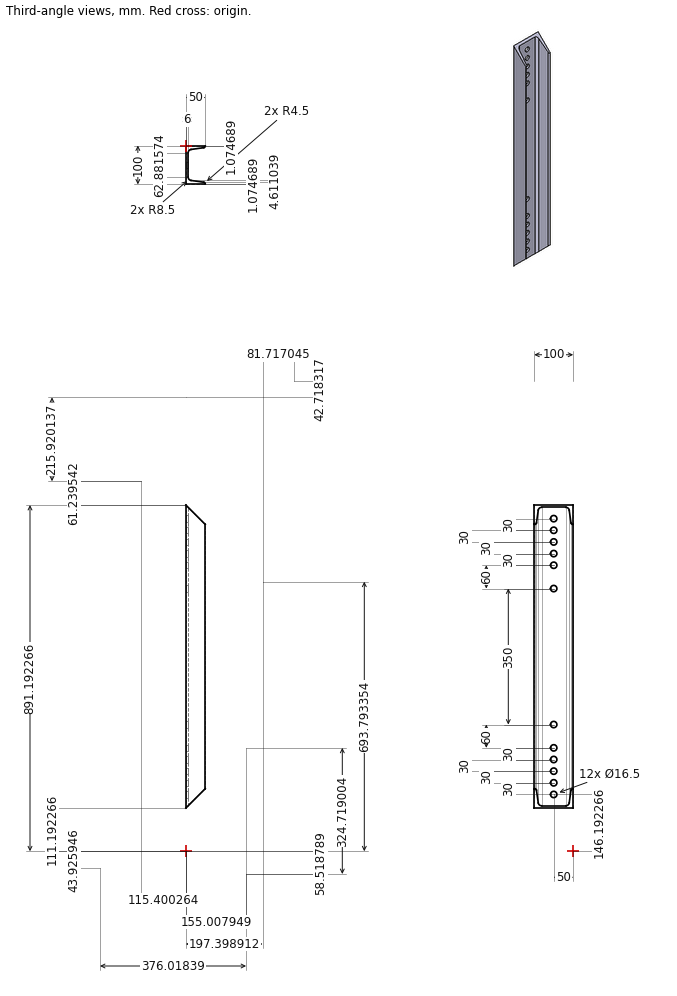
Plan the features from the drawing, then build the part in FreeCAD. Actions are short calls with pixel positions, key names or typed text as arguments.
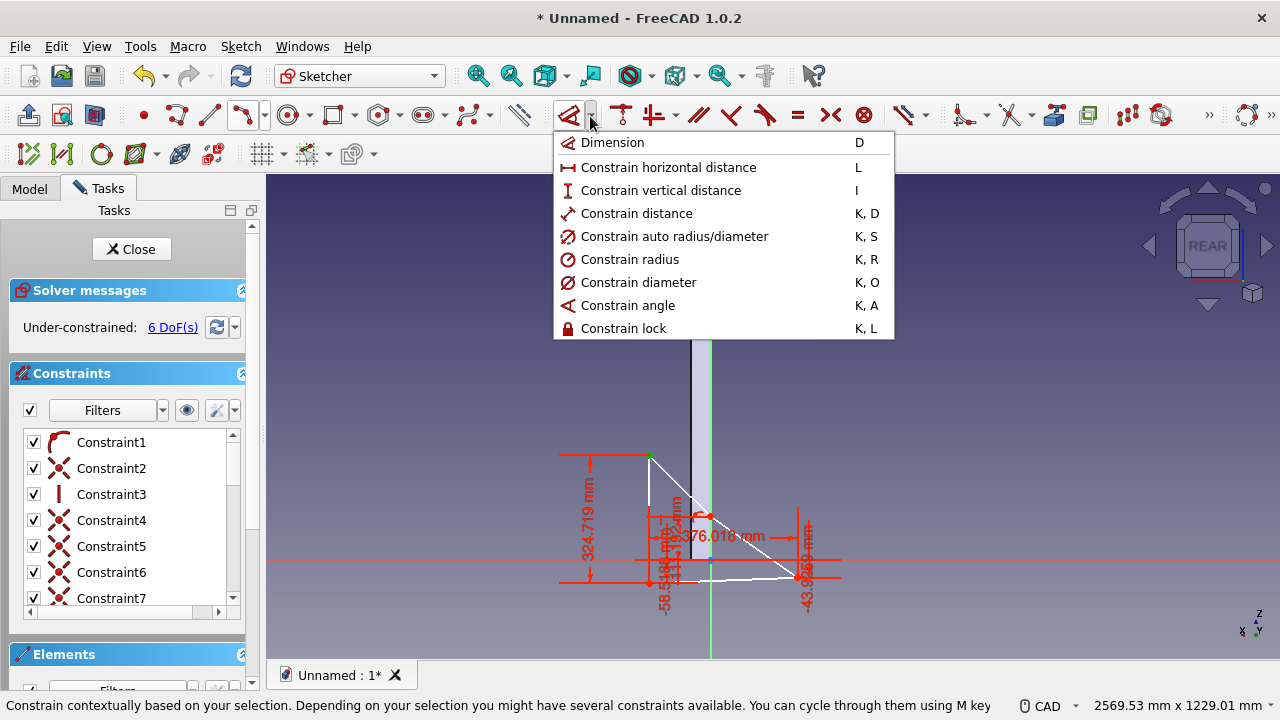
click(724, 168)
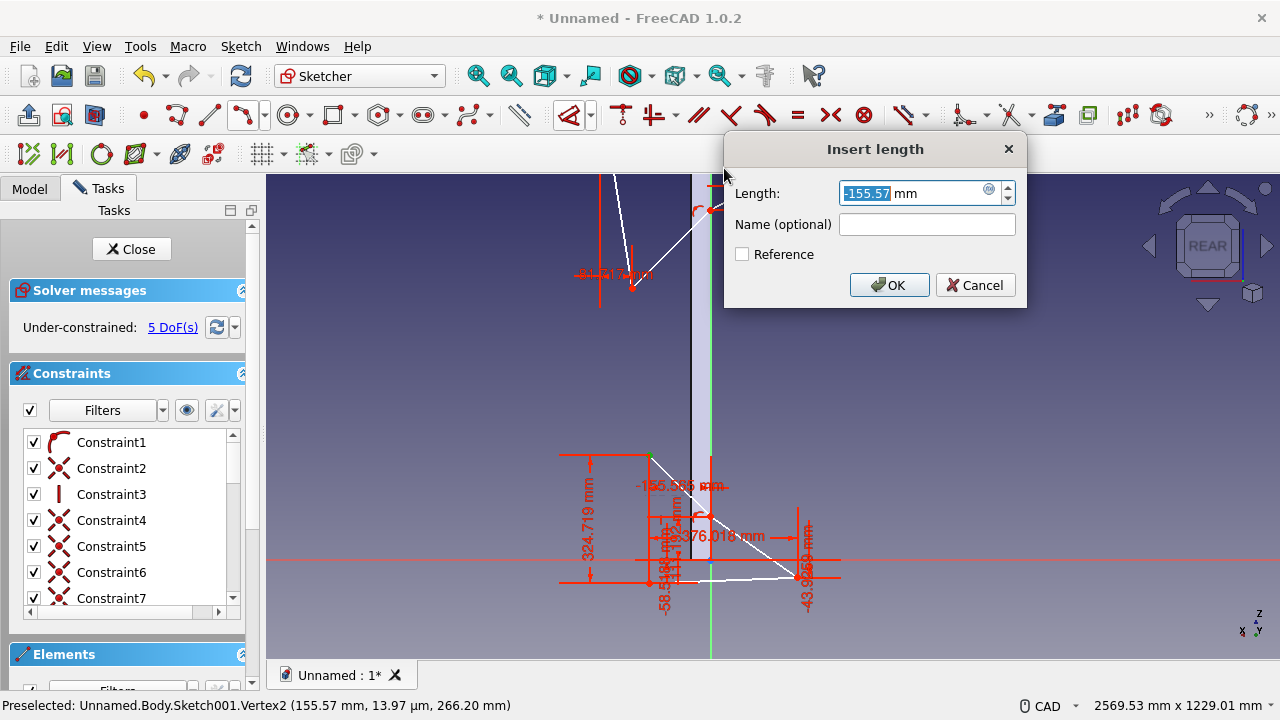
text(-155.007949)
key(Return)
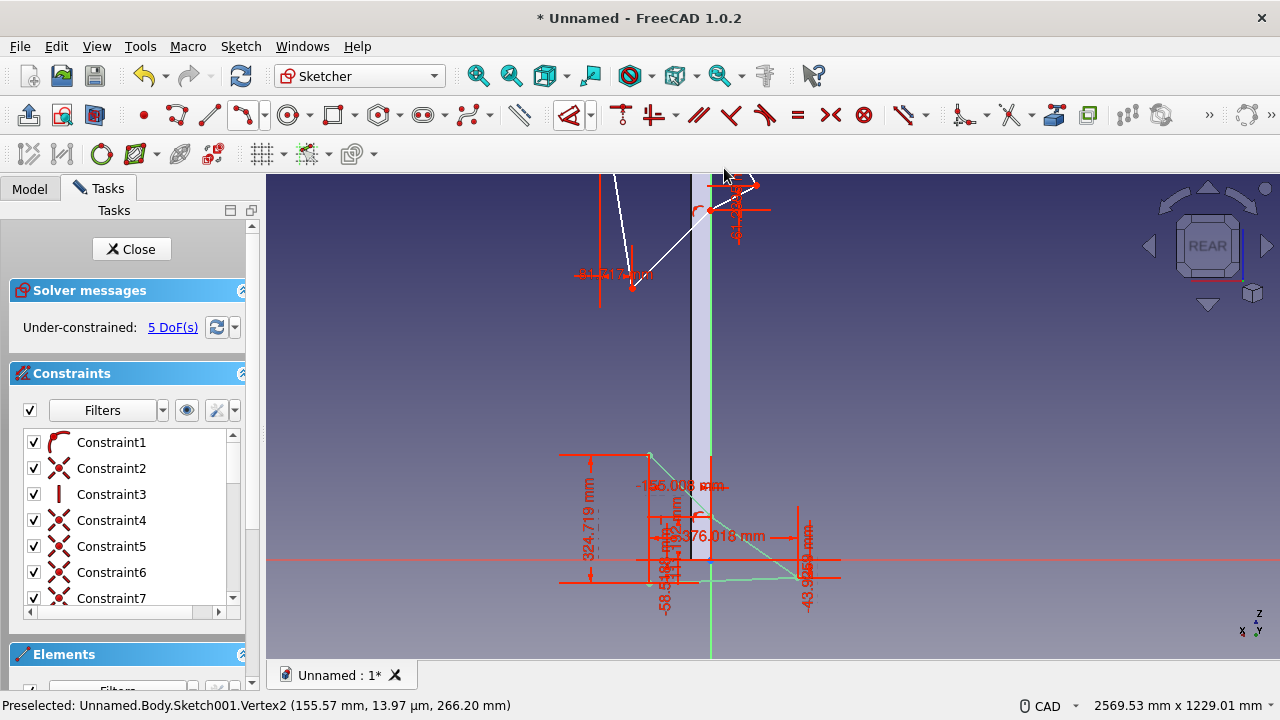
click(632, 288)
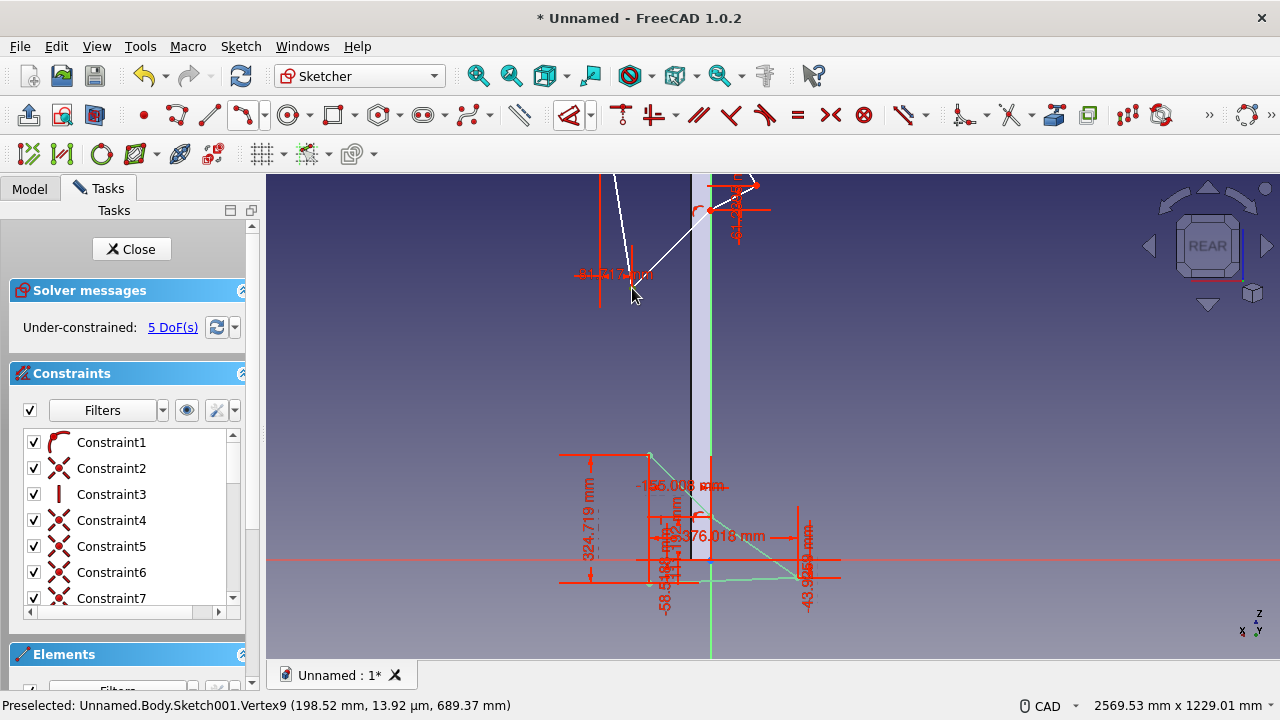
key(l)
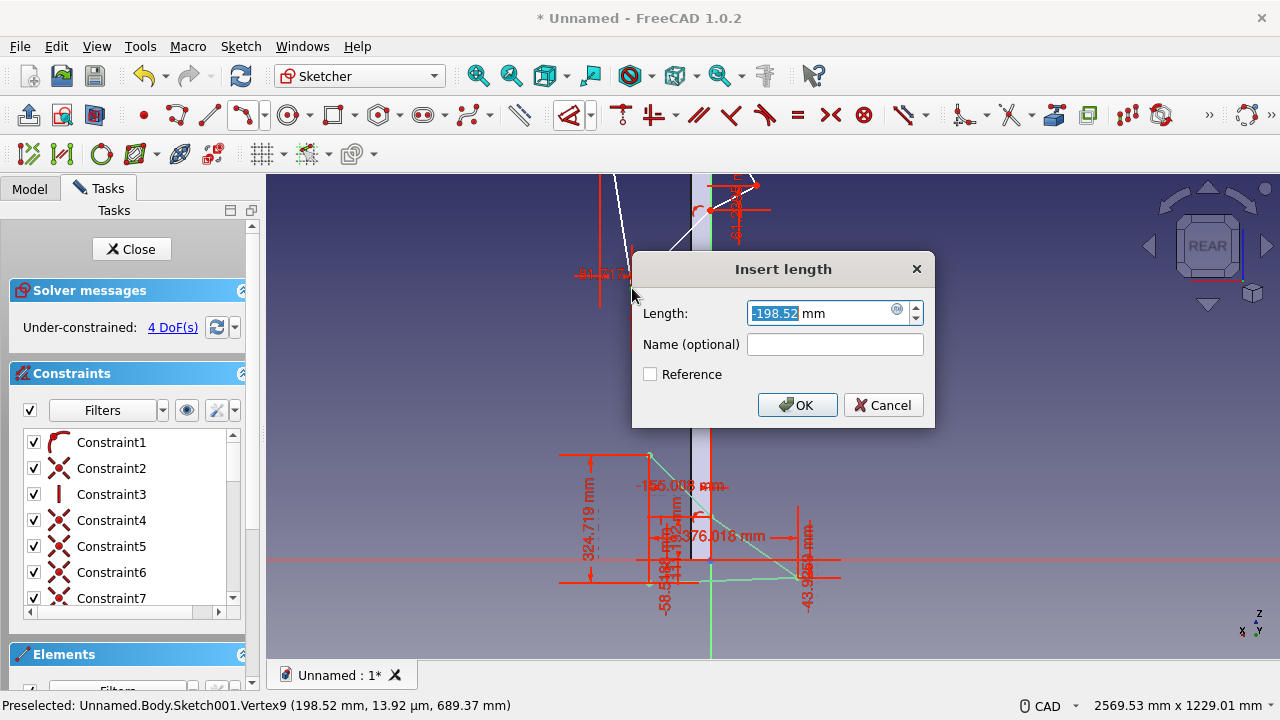
text(-197.398912)
key(Return)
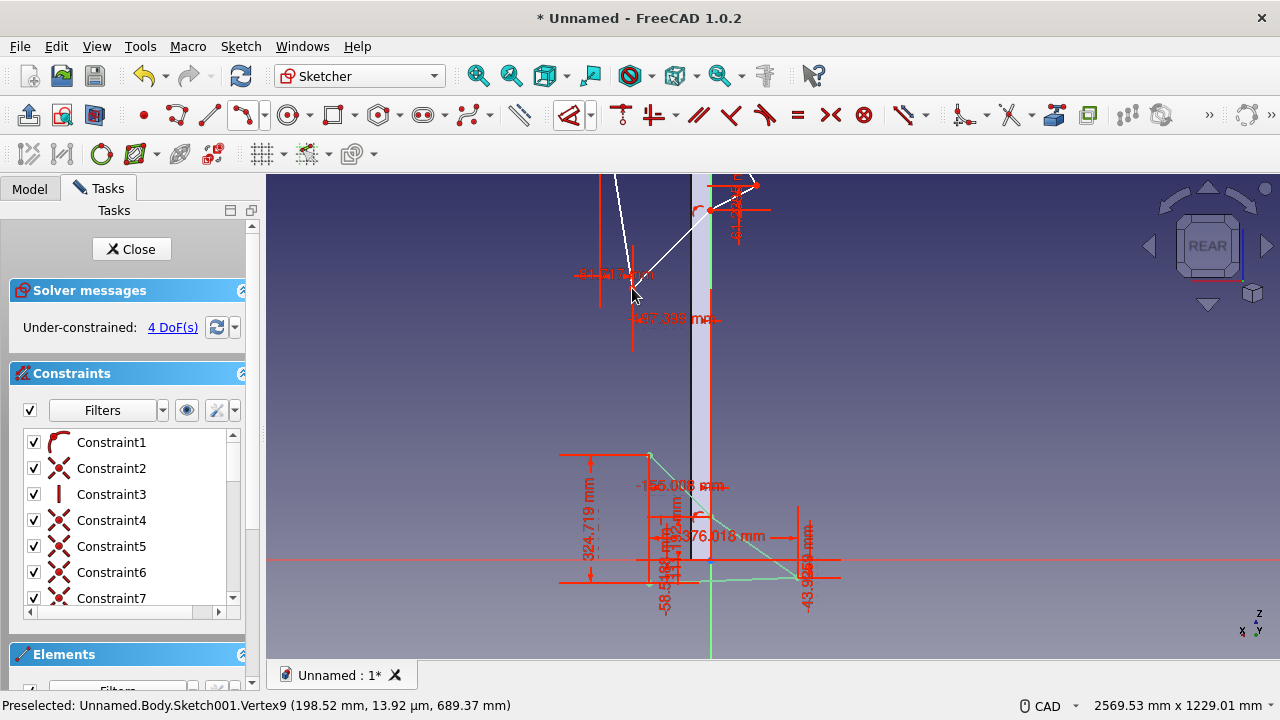
click(633, 288)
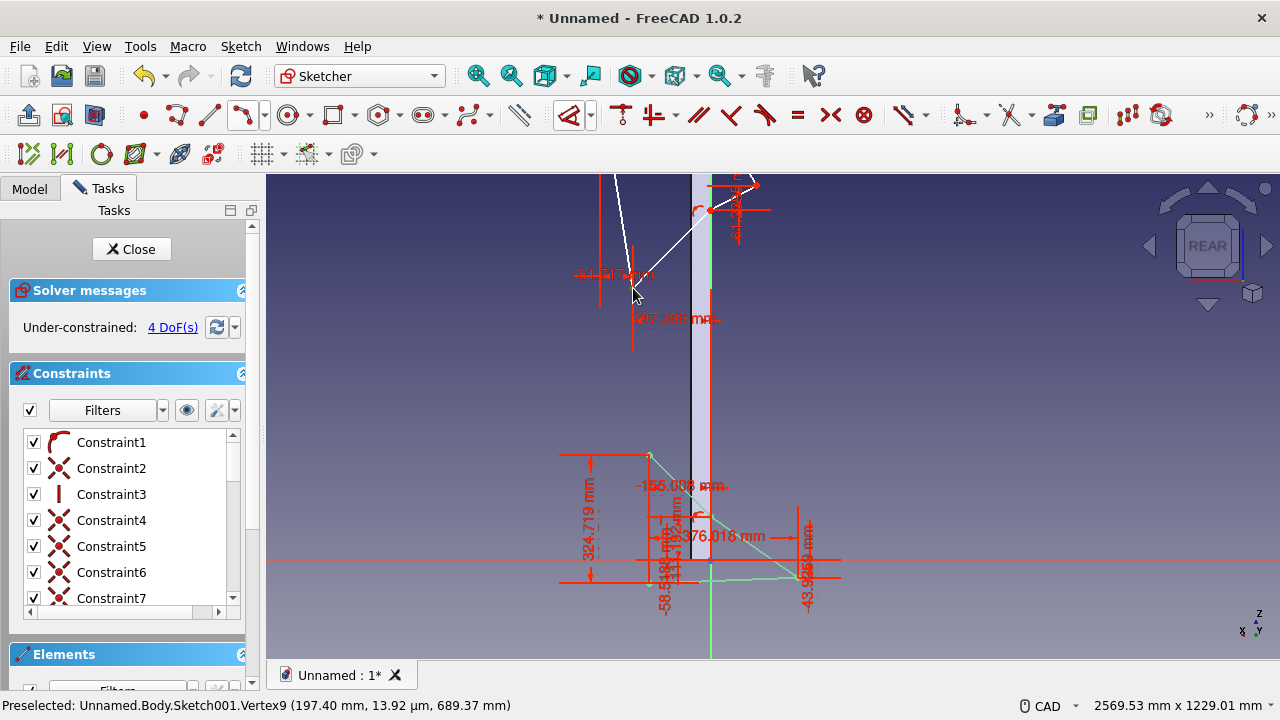
key(i)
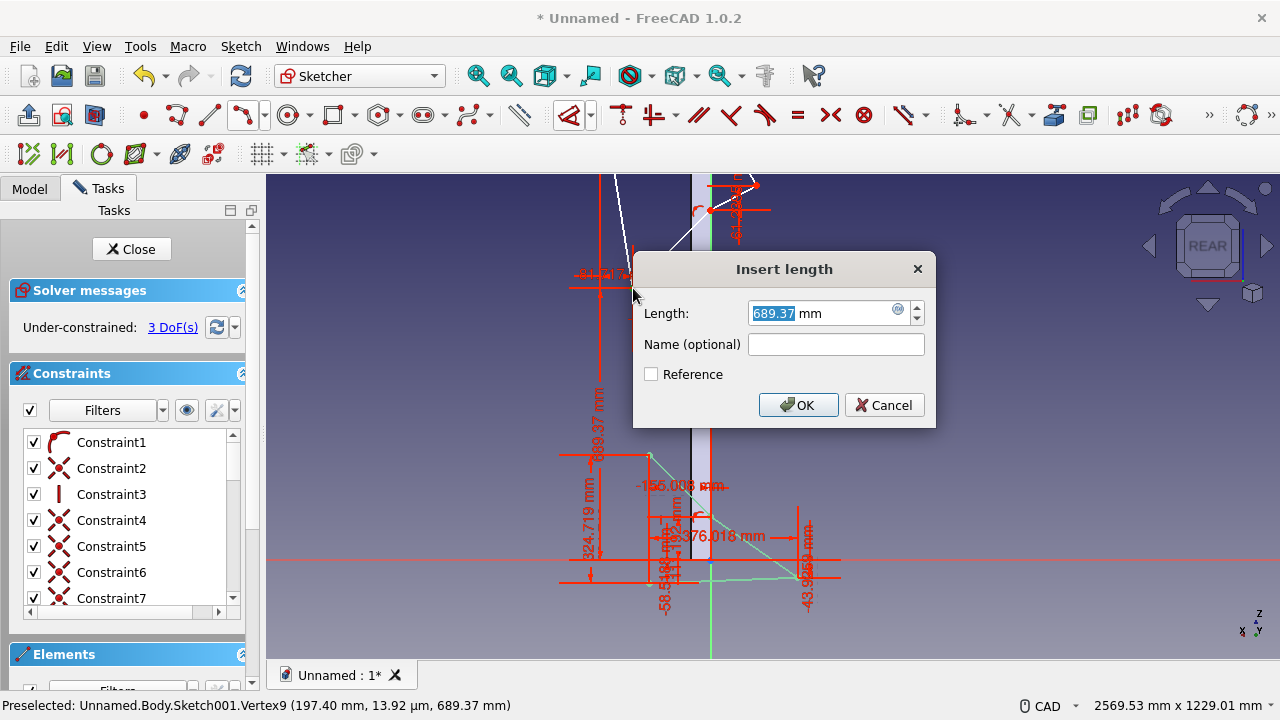
text(693.793354)
key(Return)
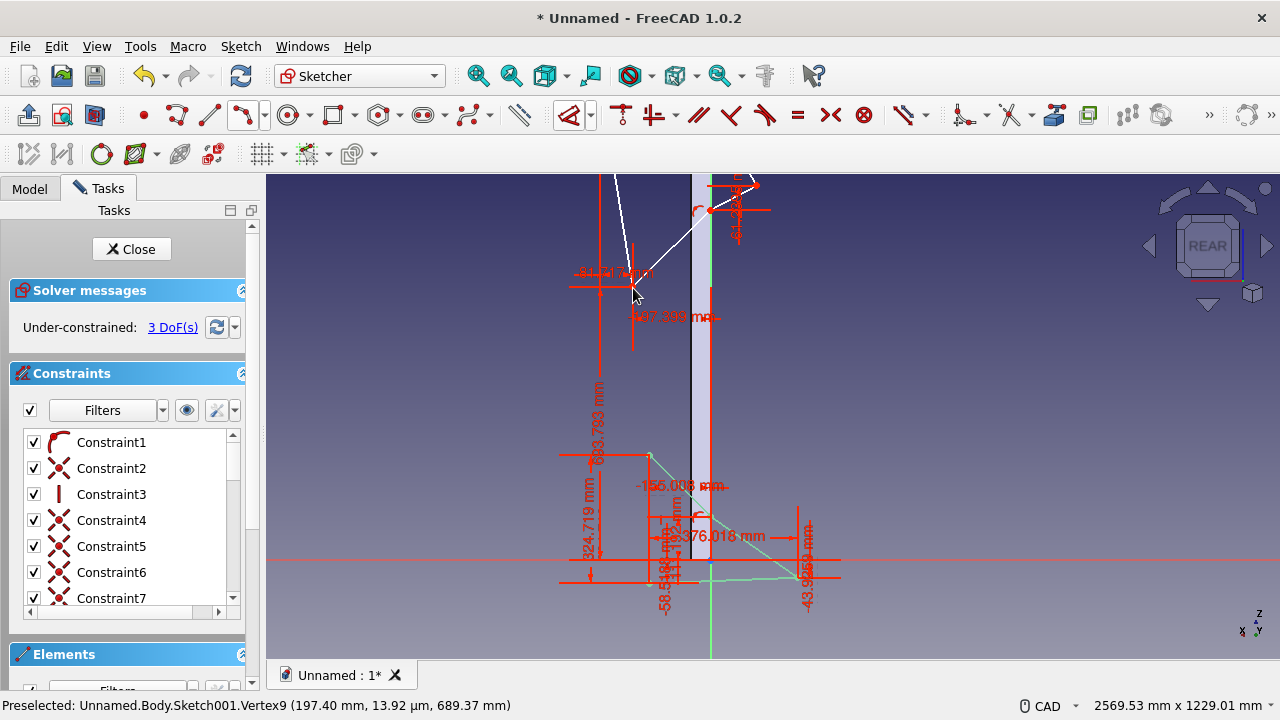
click(711, 210)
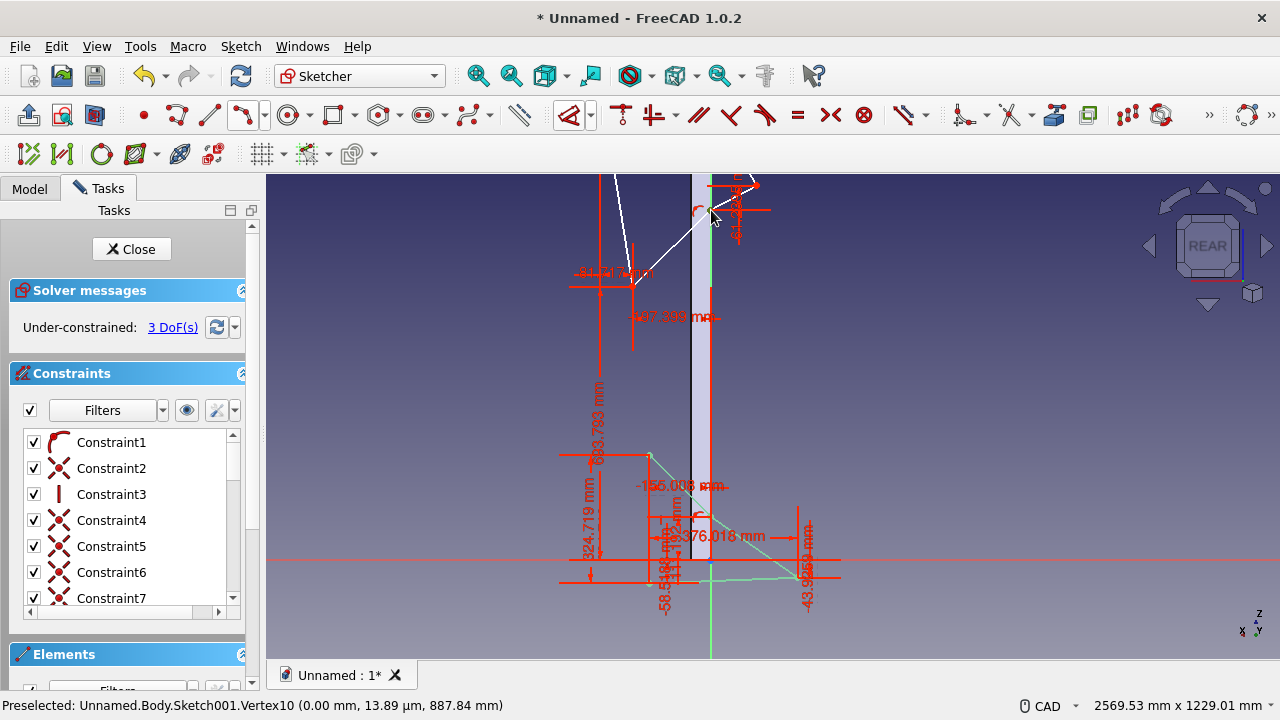
key(i)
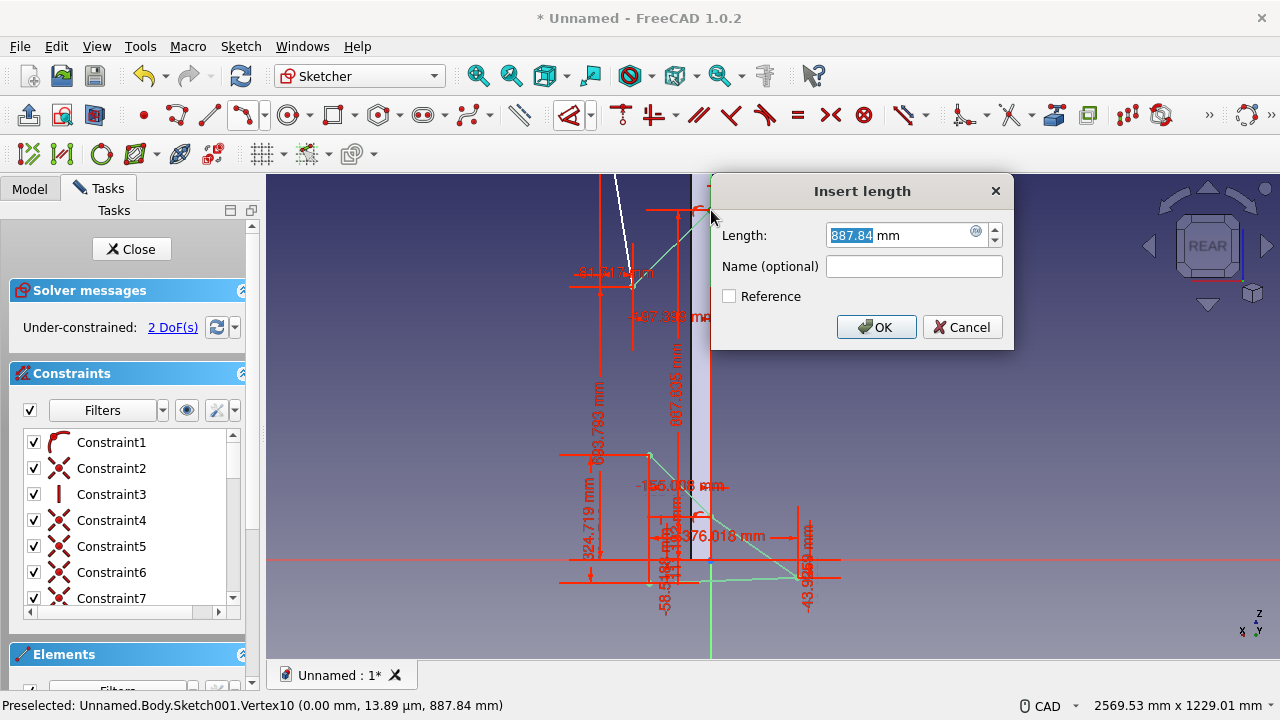
text(891.192266)
key(Return)